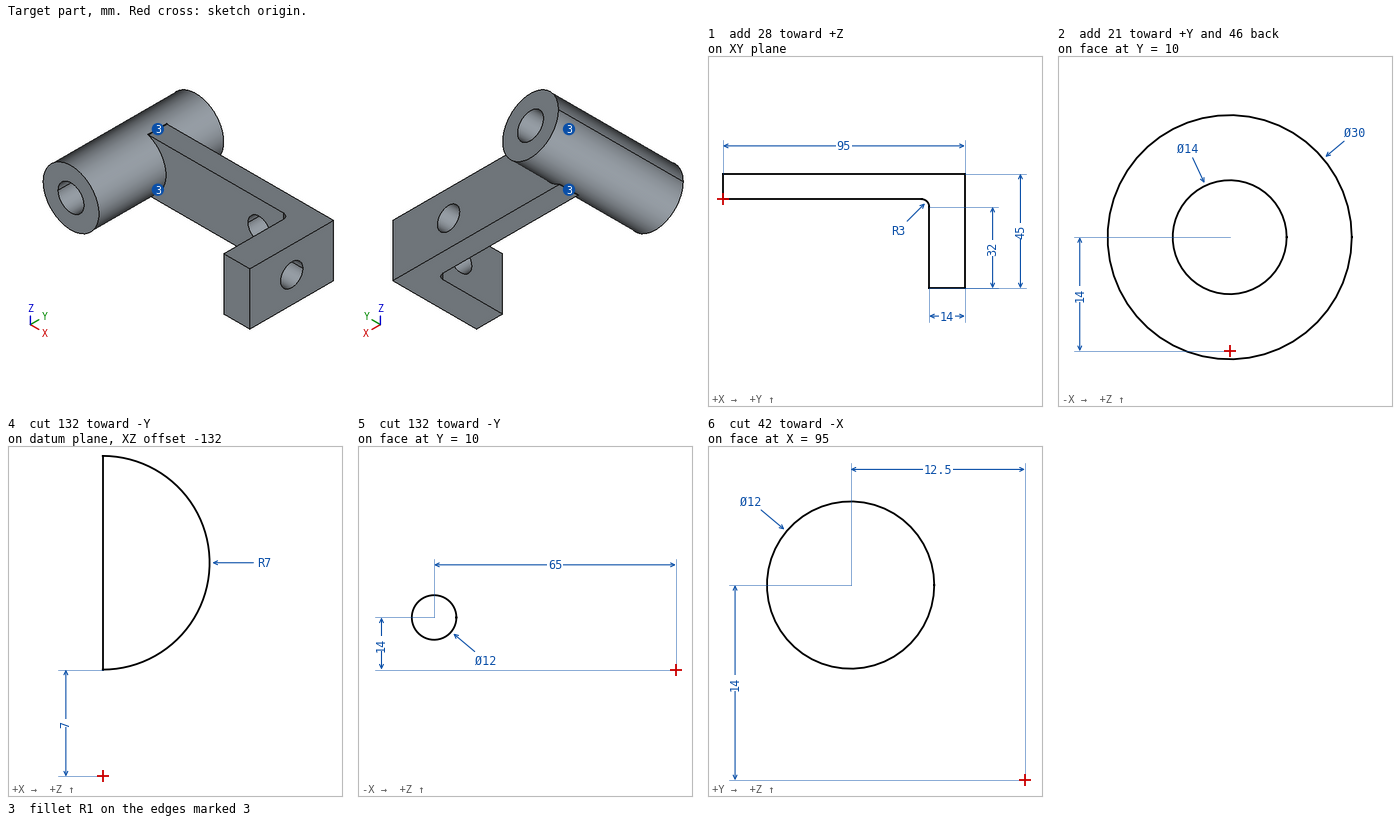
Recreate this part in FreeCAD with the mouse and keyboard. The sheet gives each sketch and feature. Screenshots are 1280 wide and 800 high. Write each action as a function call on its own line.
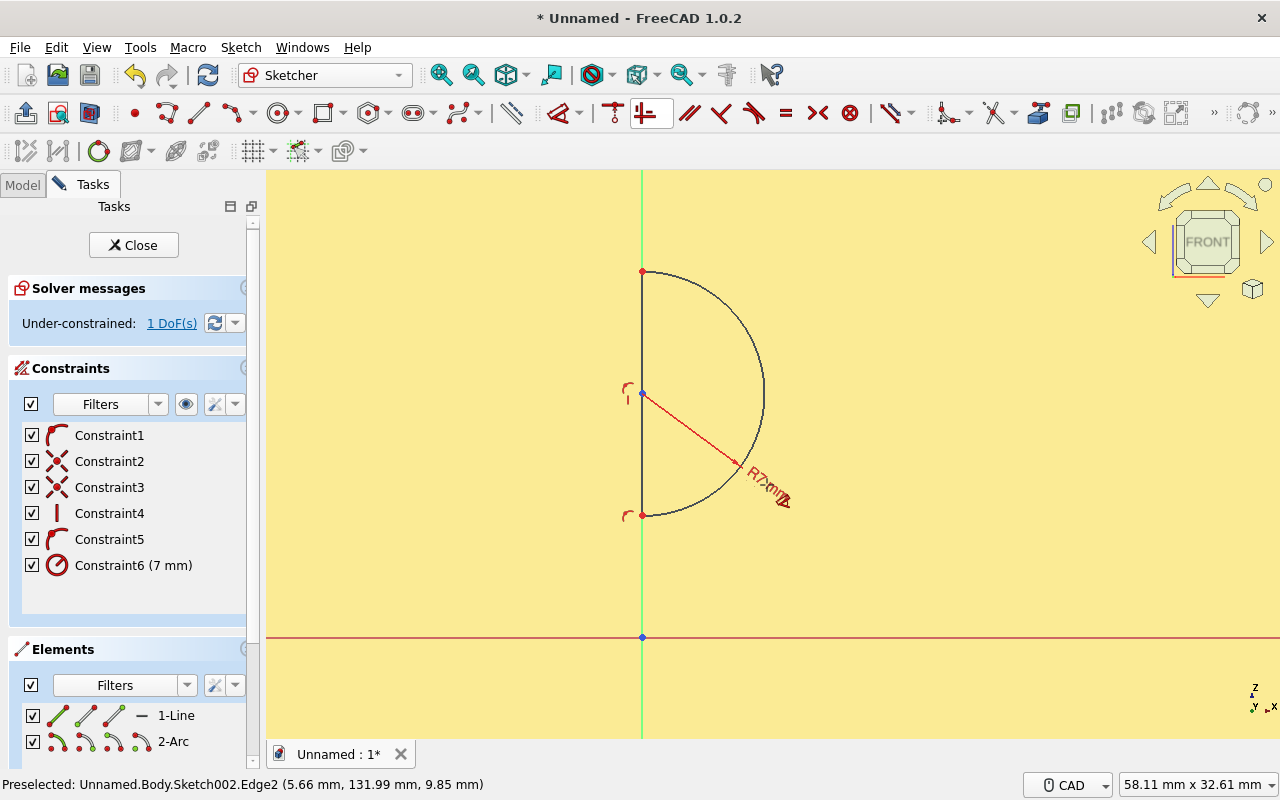
click(642, 516)
click(608, 577)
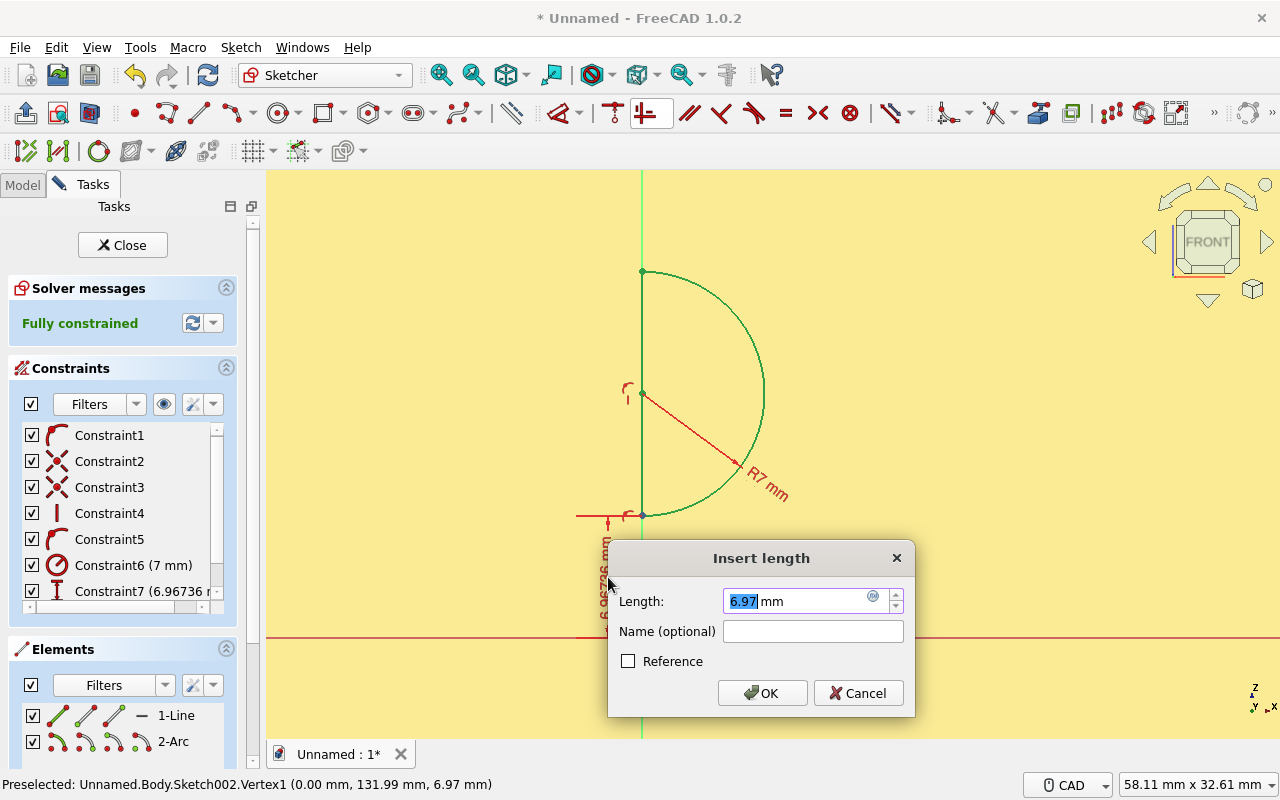
text(7)
key(Return)
key(Escape)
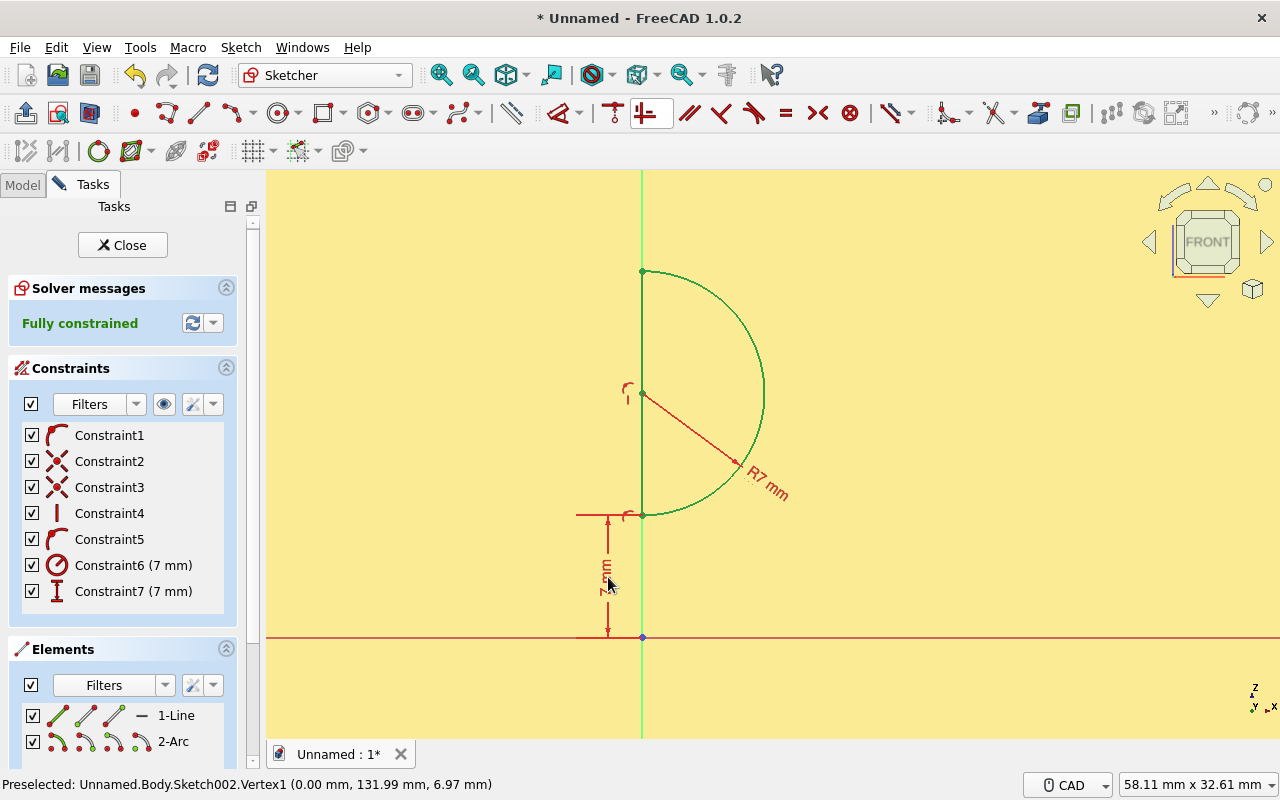
click(123, 245)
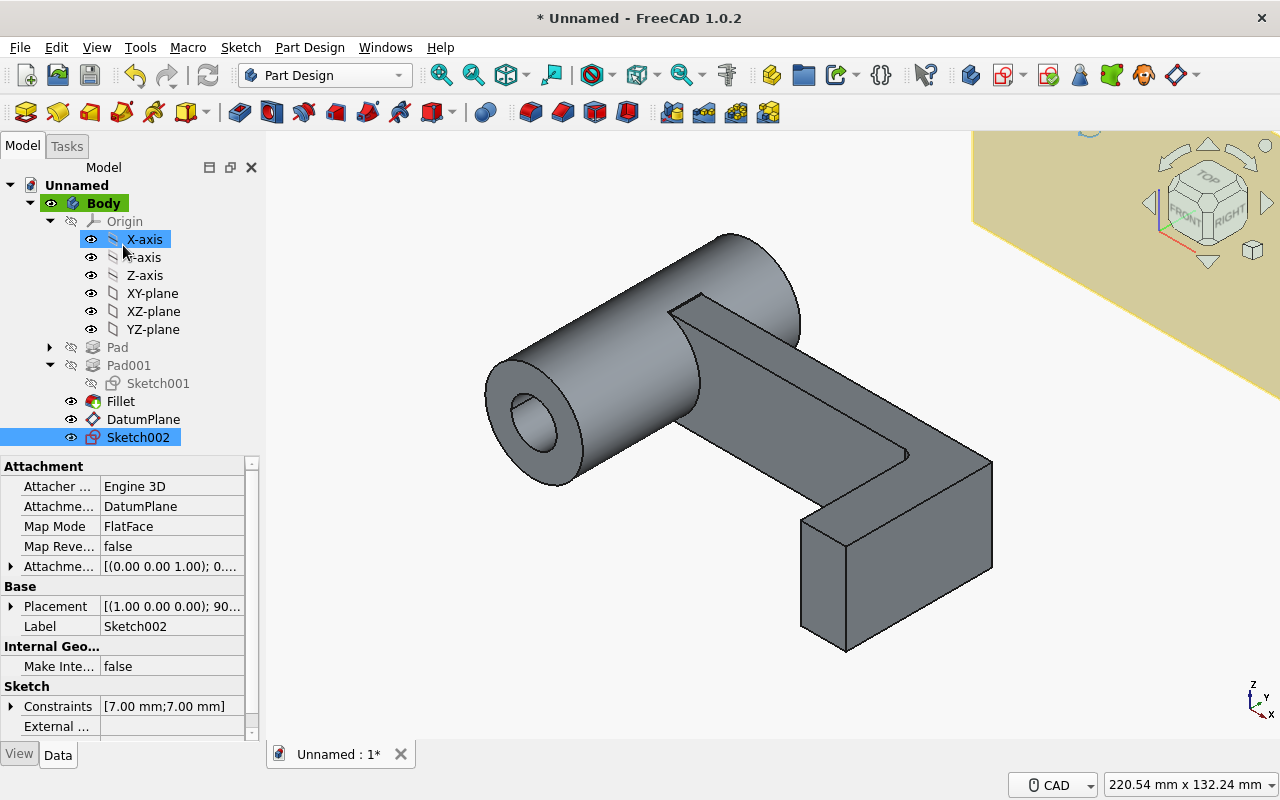
click(240, 112)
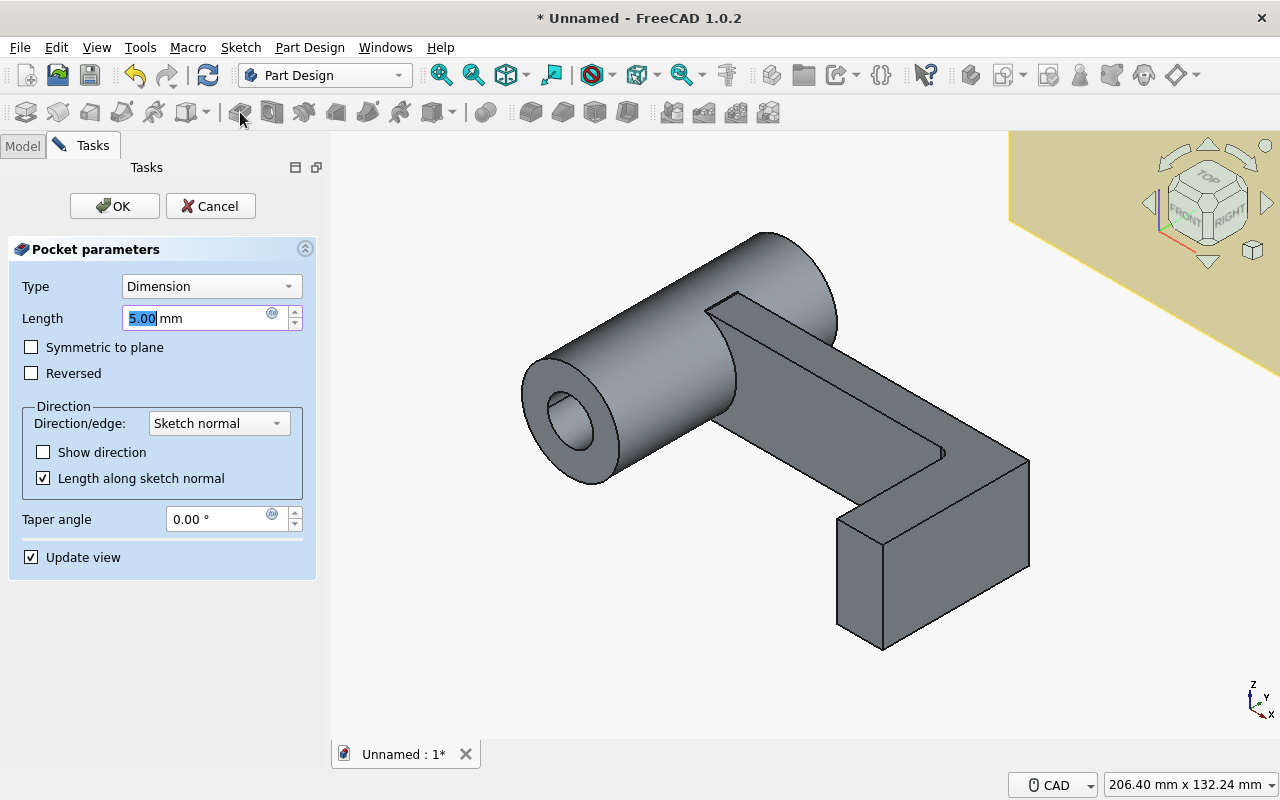
text(132)
key(Tab)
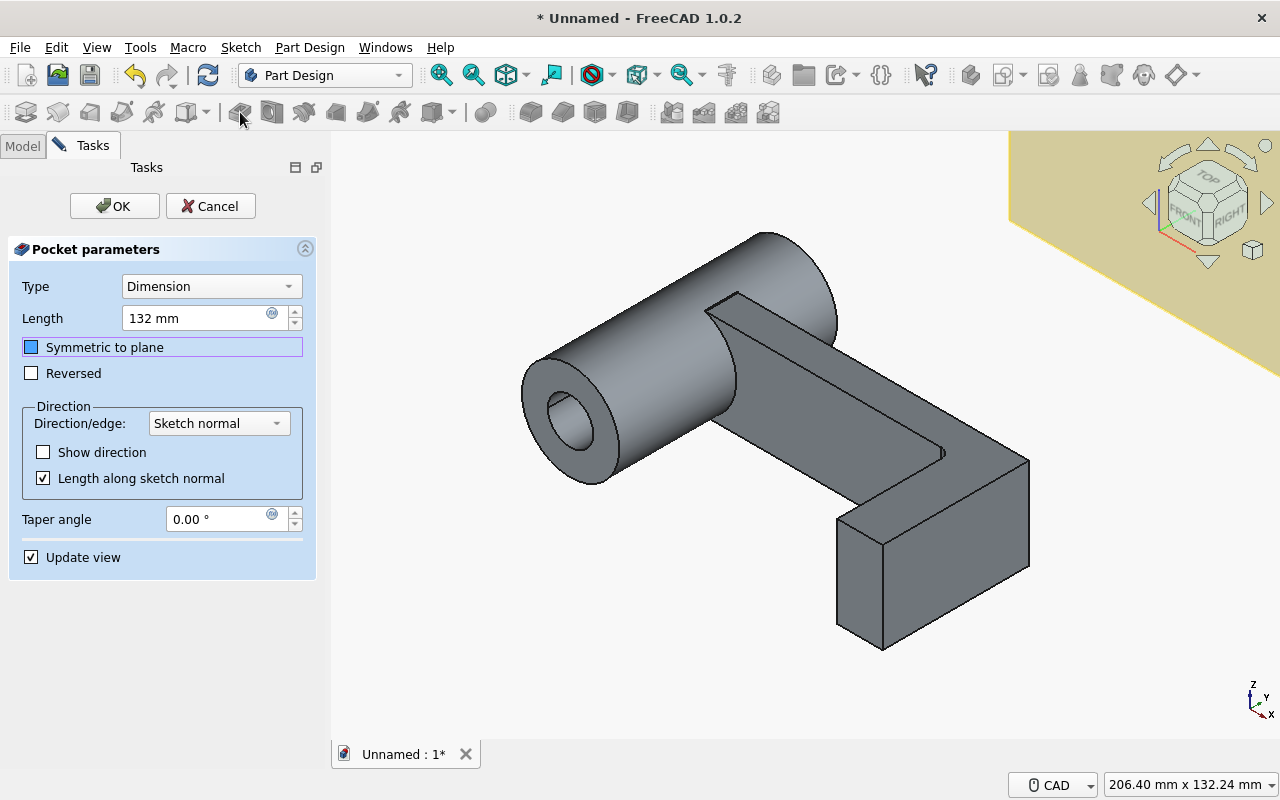
click(30, 373)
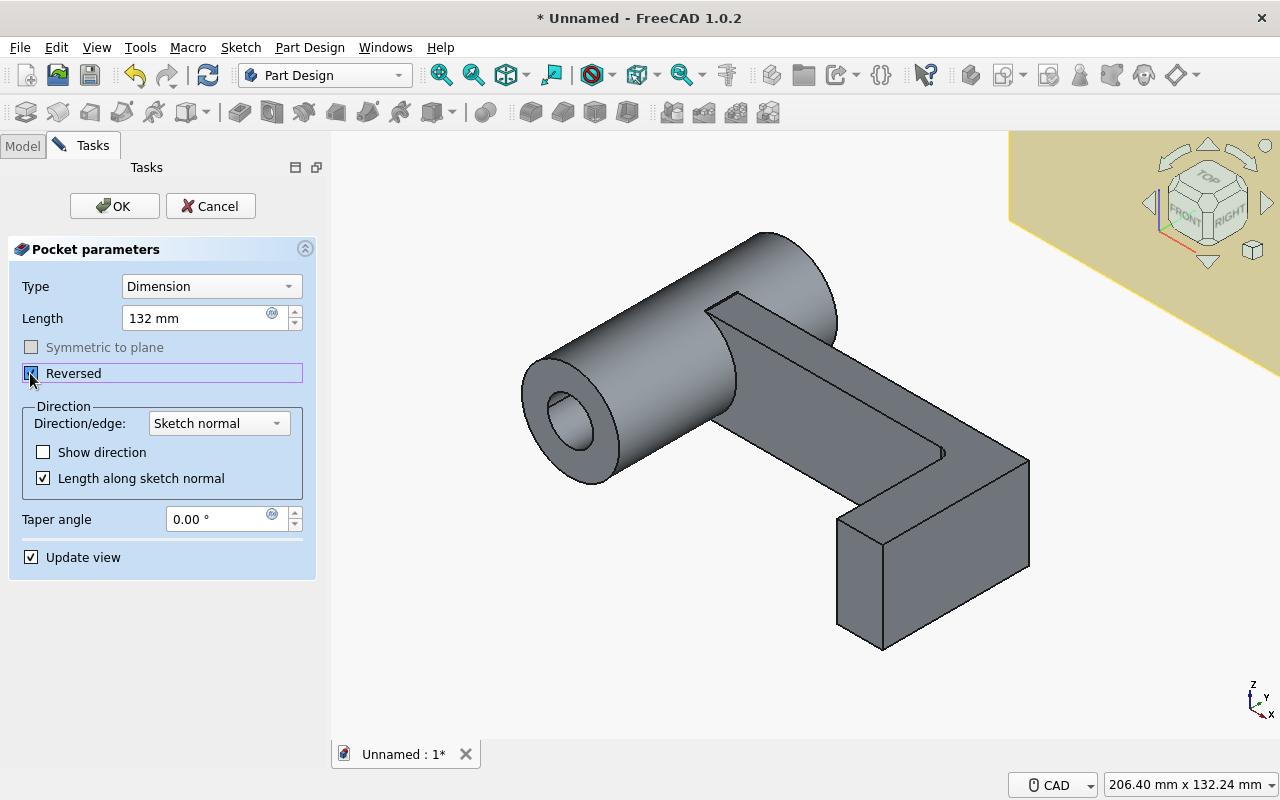
click(115, 206)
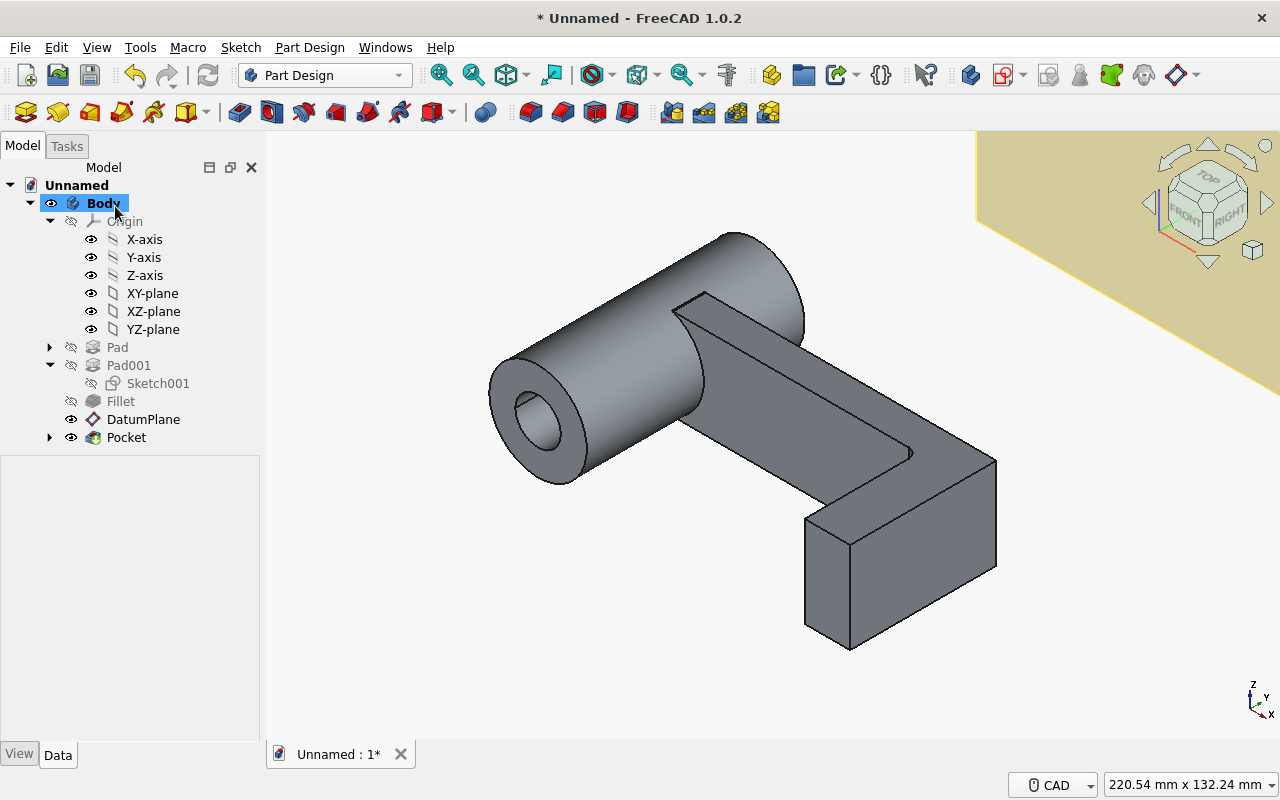
click(116, 419)
key(space)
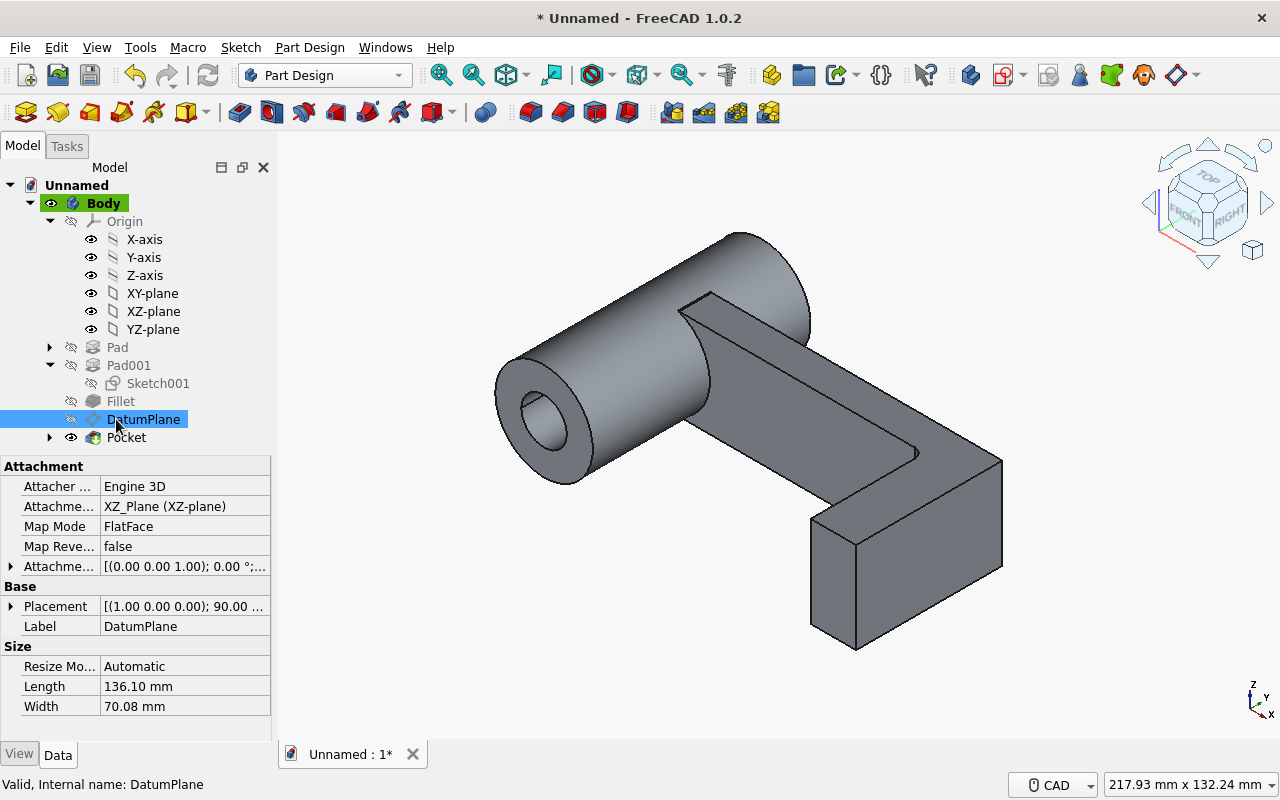
key(4)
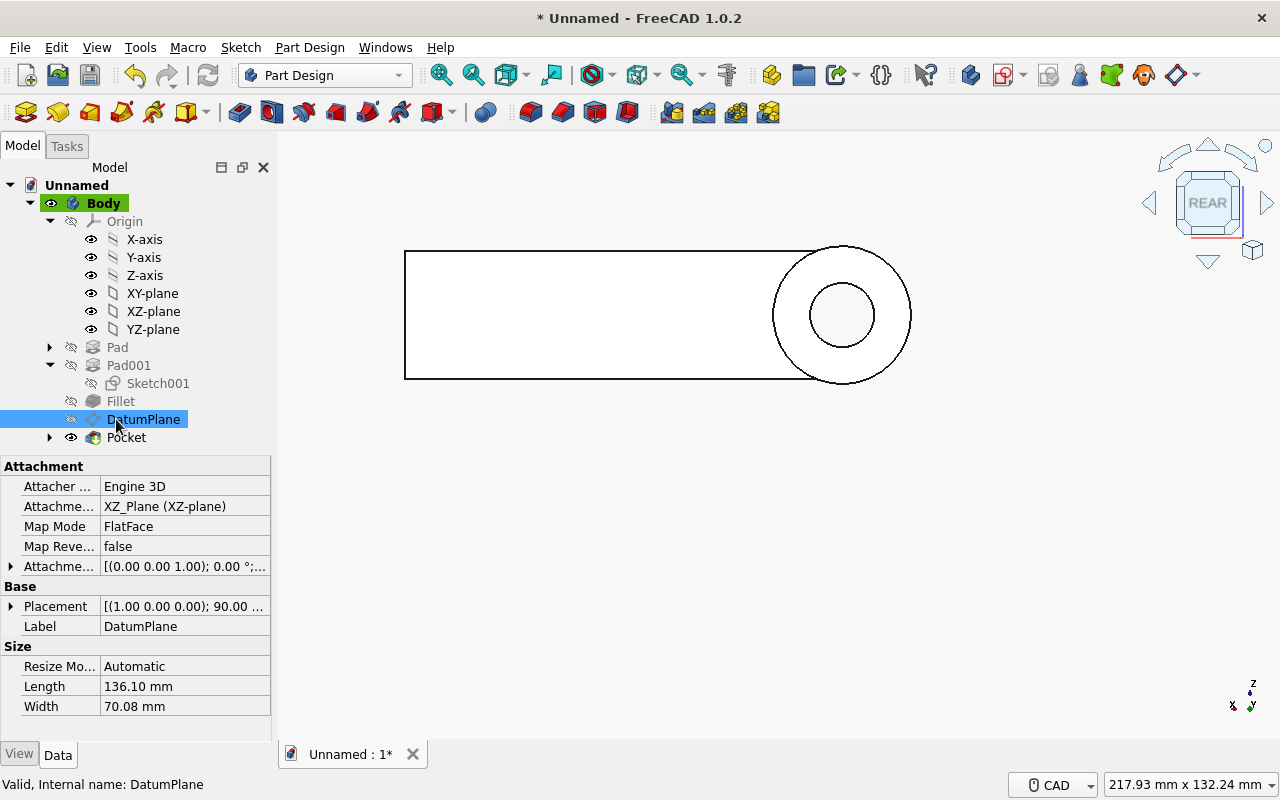
click(494, 314)